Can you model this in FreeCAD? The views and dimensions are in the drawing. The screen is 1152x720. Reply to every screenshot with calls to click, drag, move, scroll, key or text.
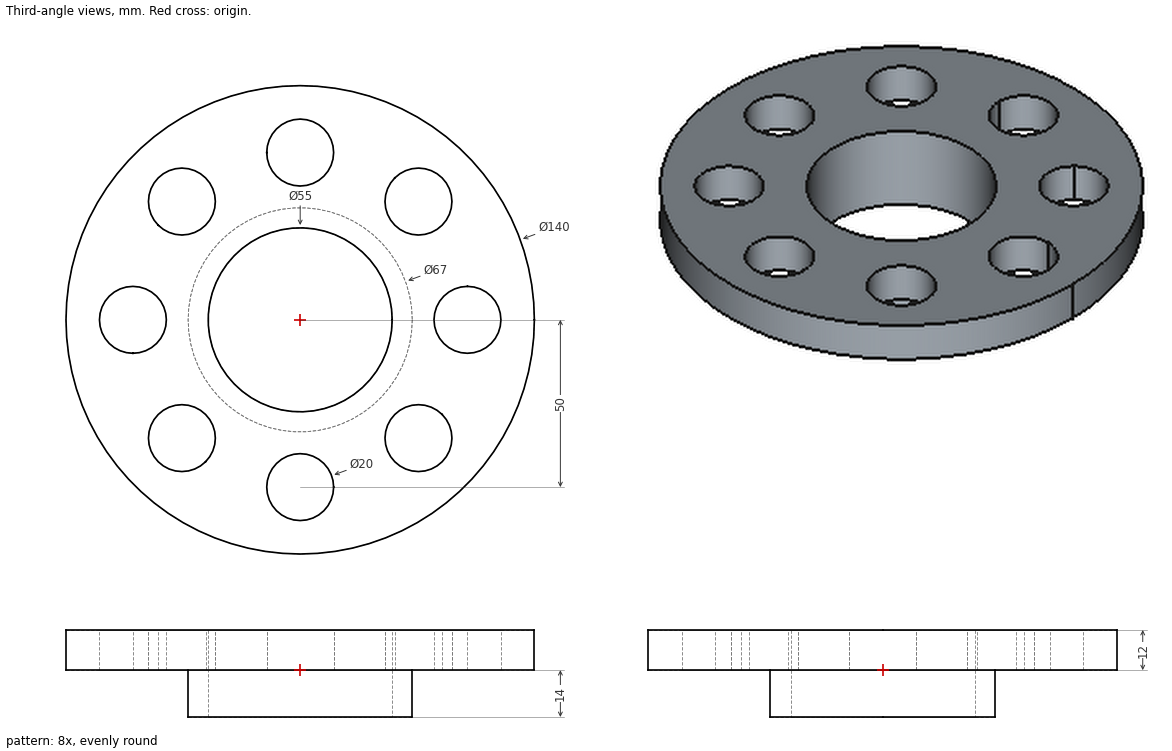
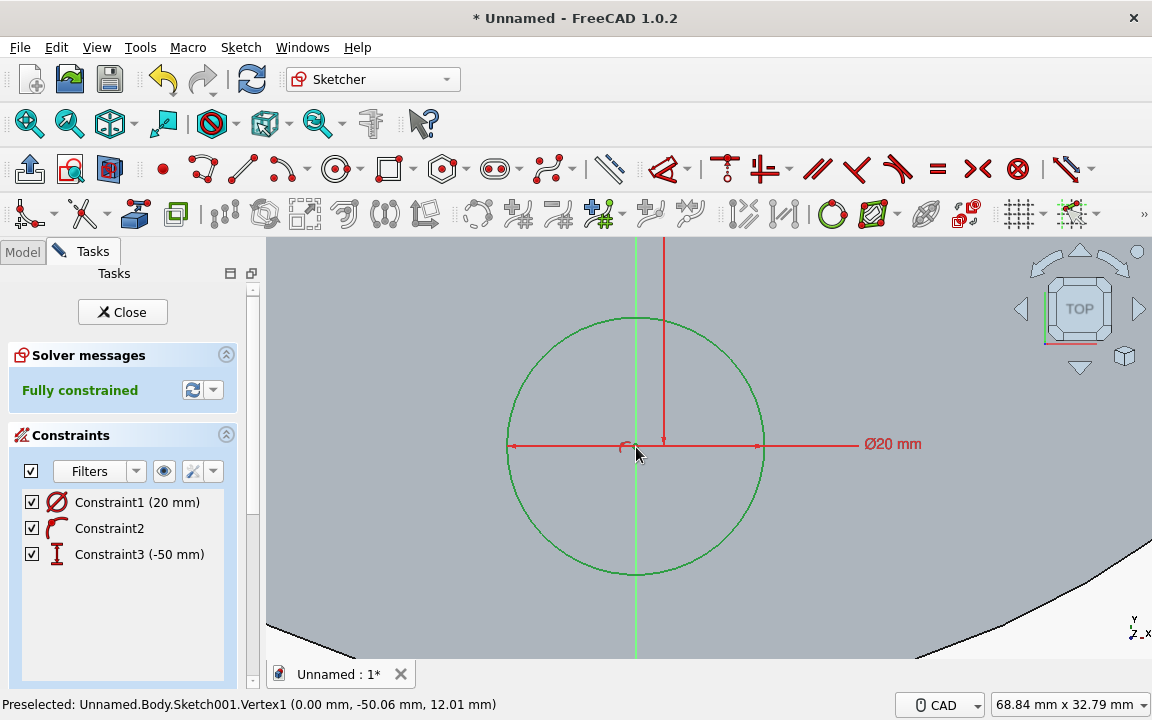
click(123, 312)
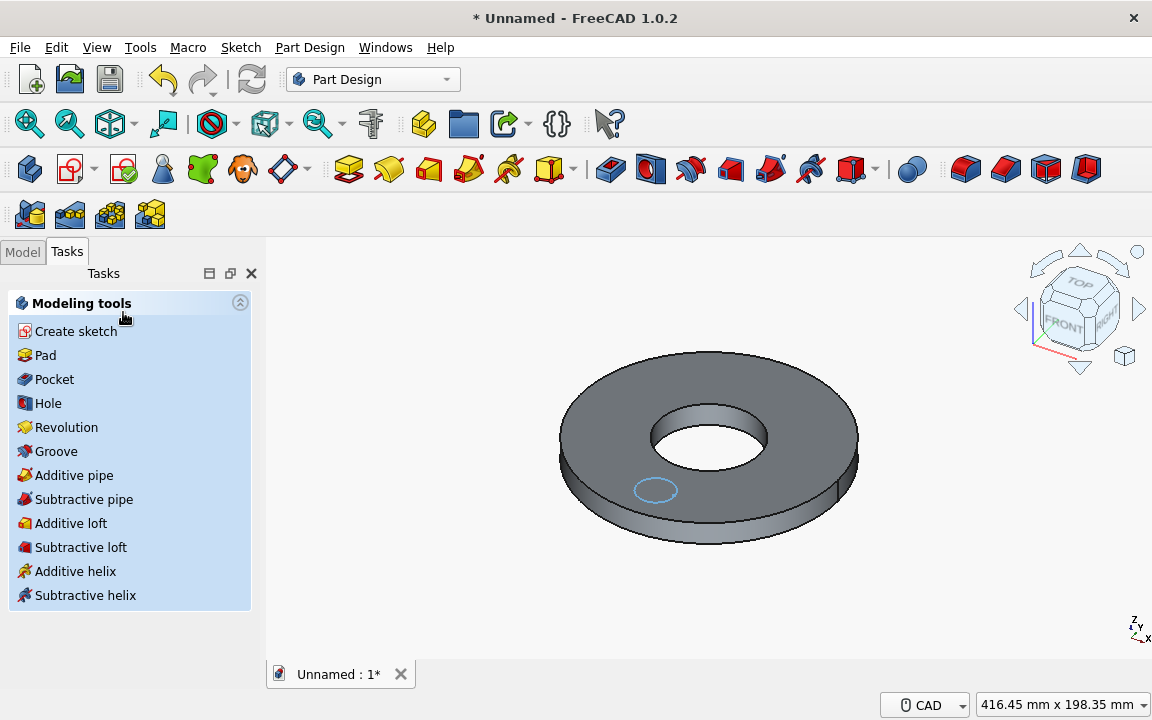
click(612, 170)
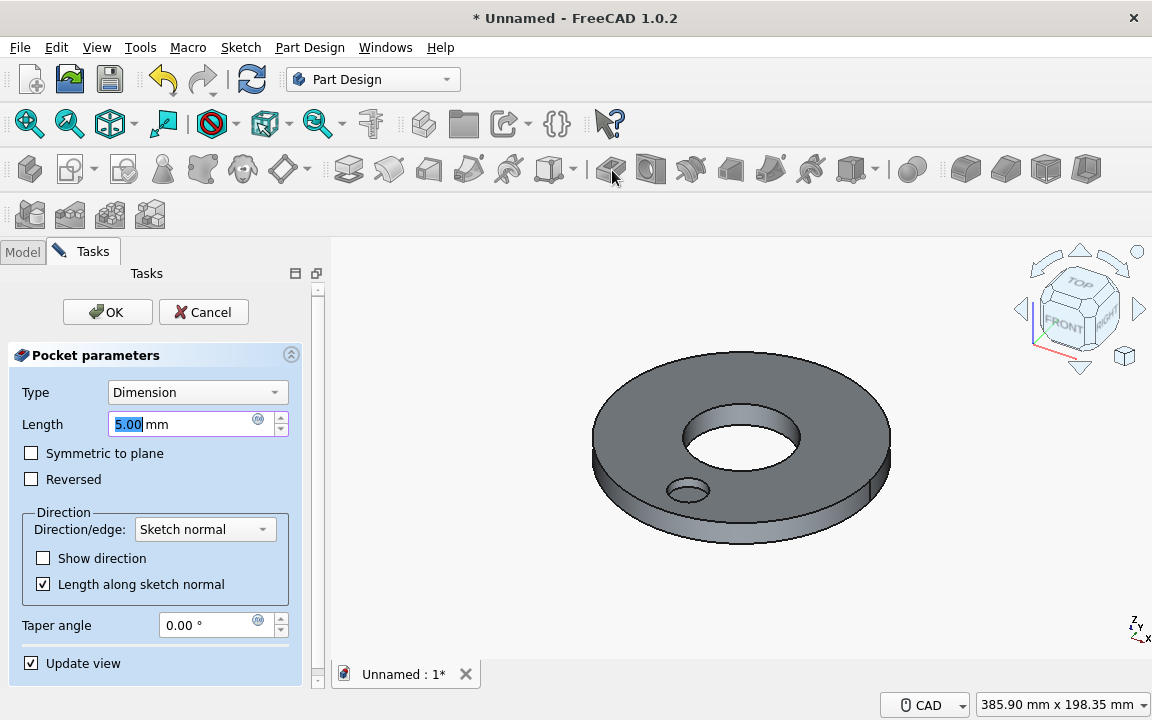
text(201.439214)
key(Tab)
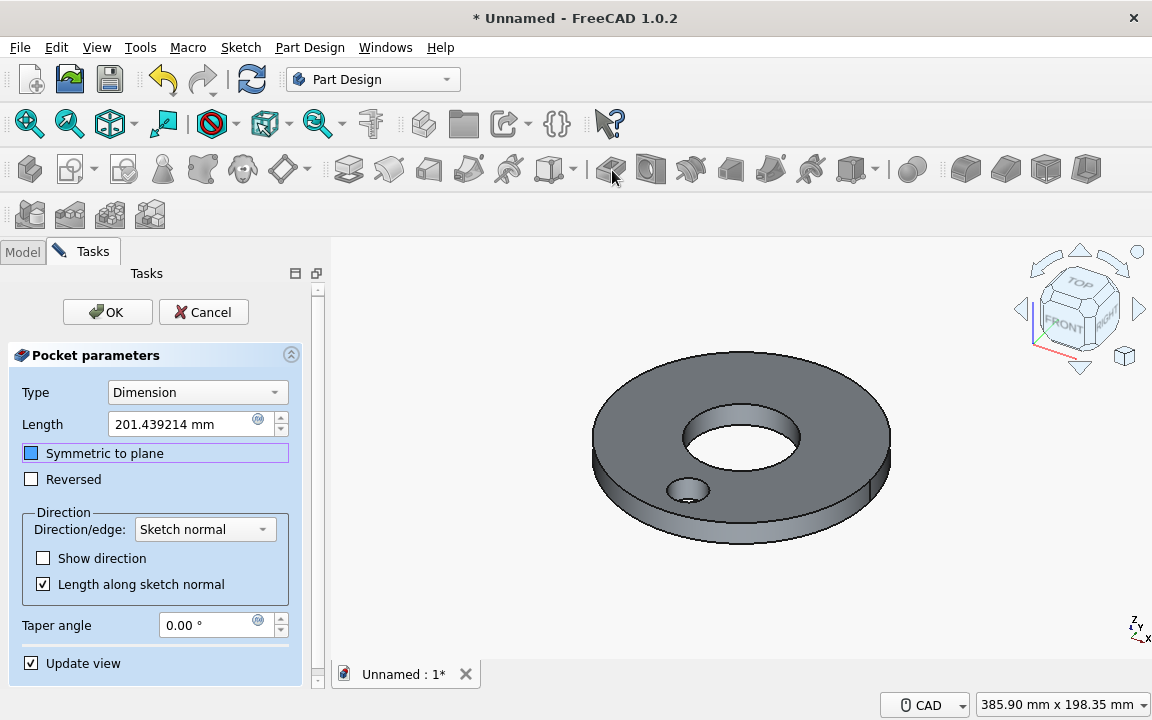
click(30, 453)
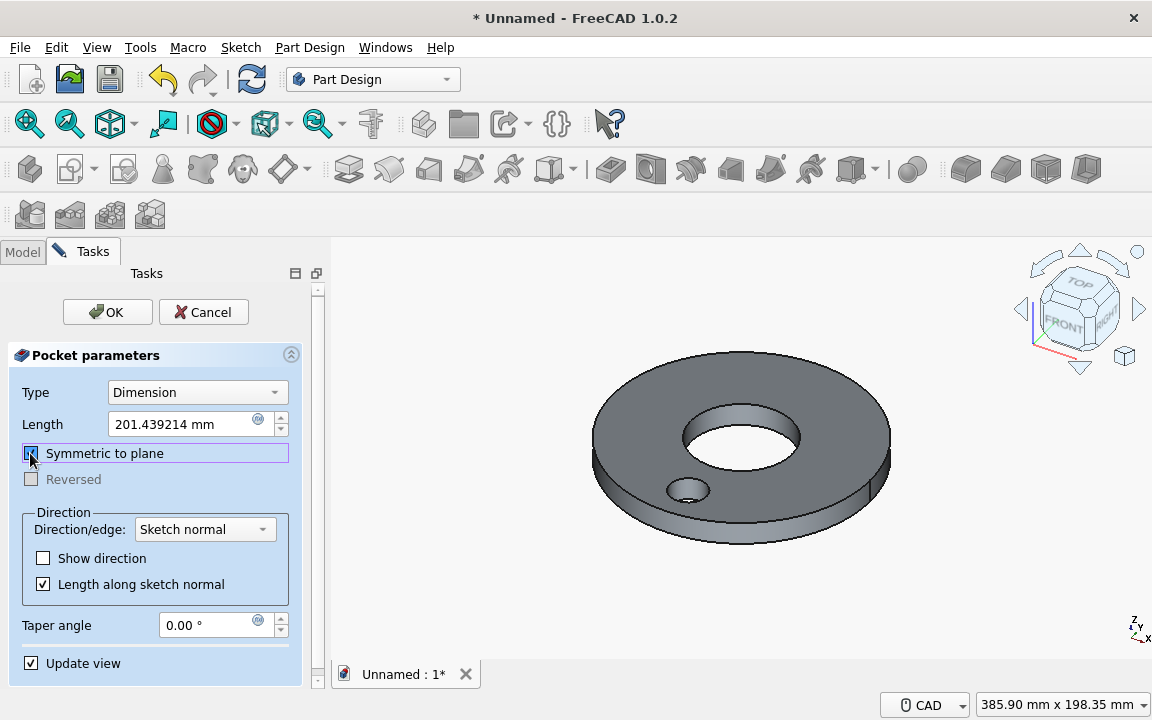
click(108, 312)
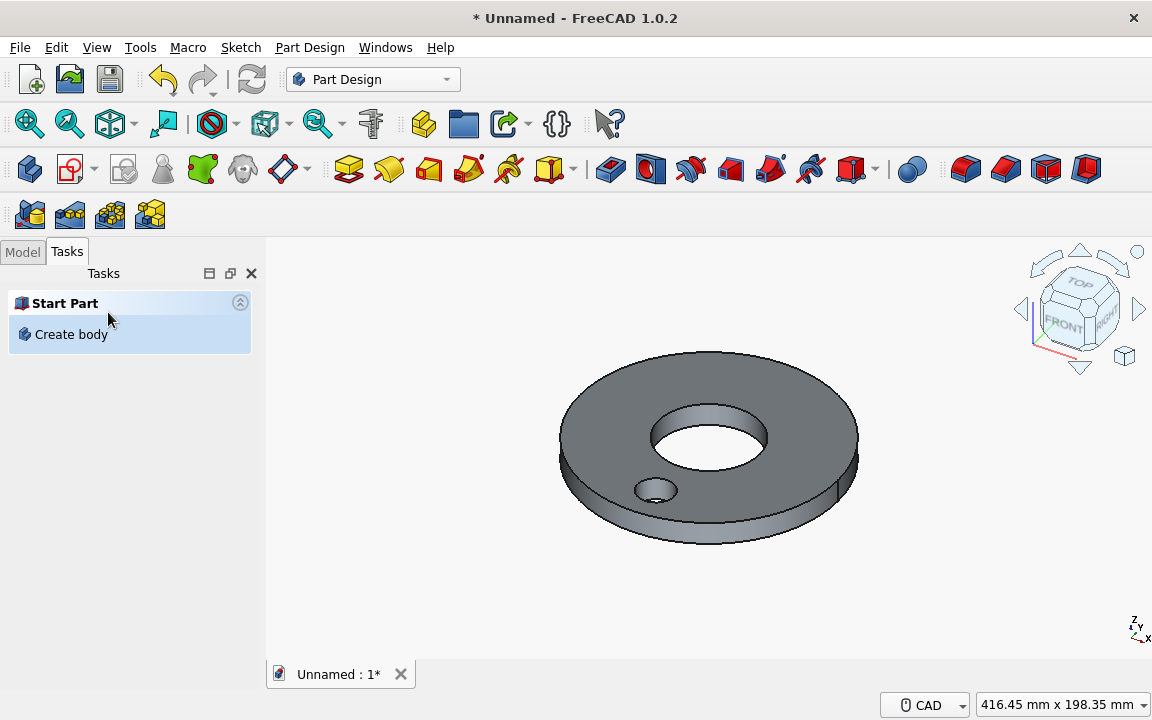
click(23, 251)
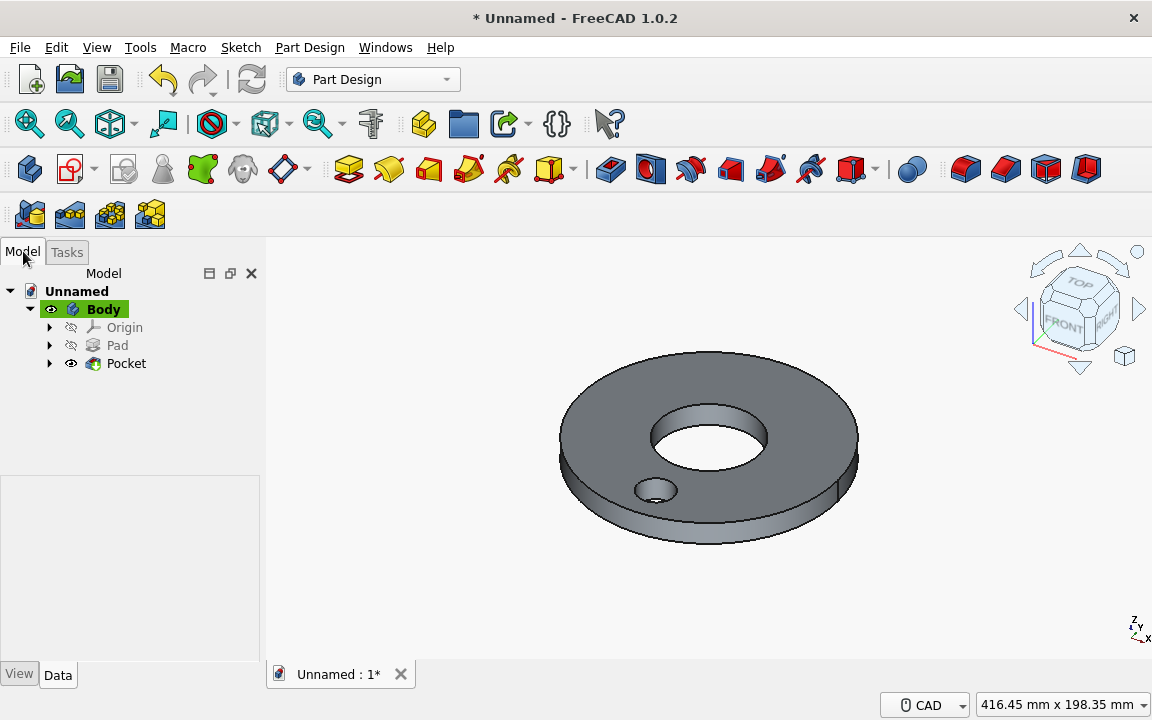
click(116, 363)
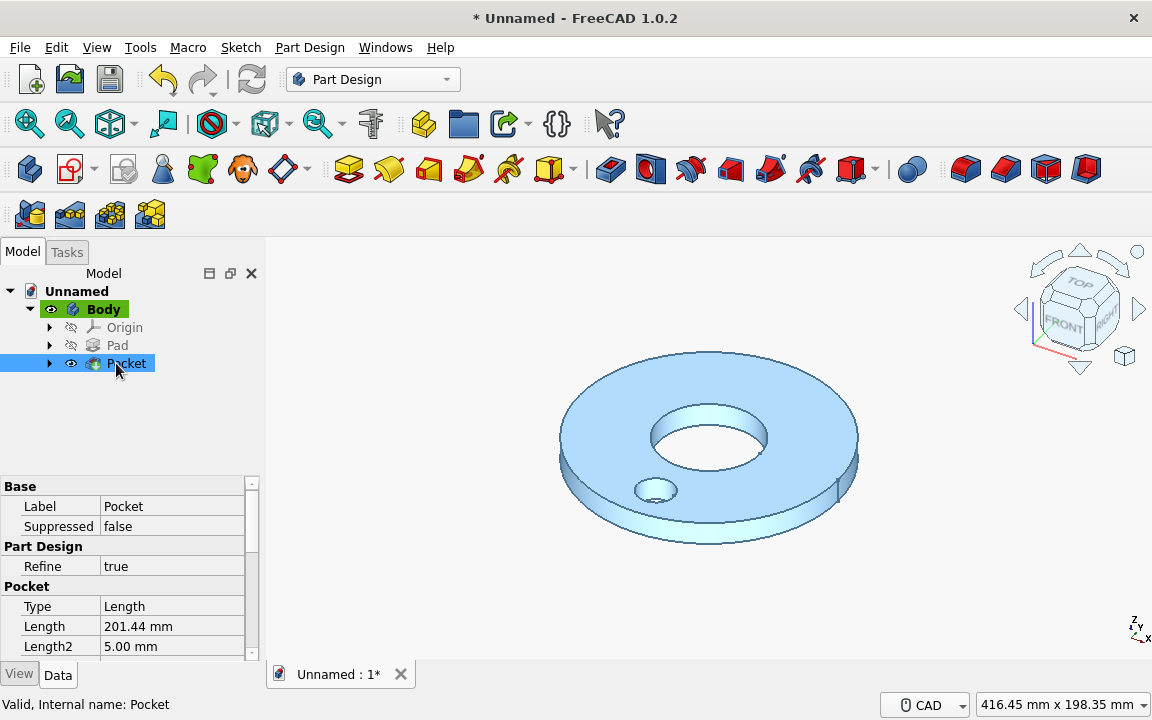
click(110, 214)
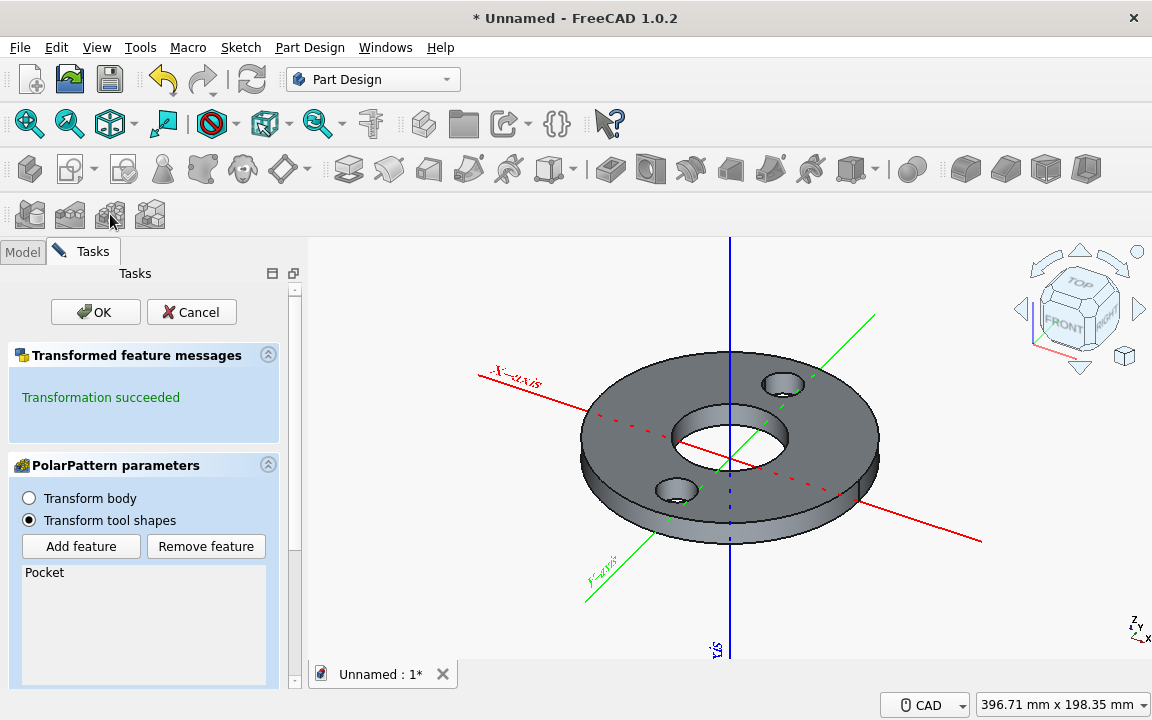
scroll(295, 486, down, 2)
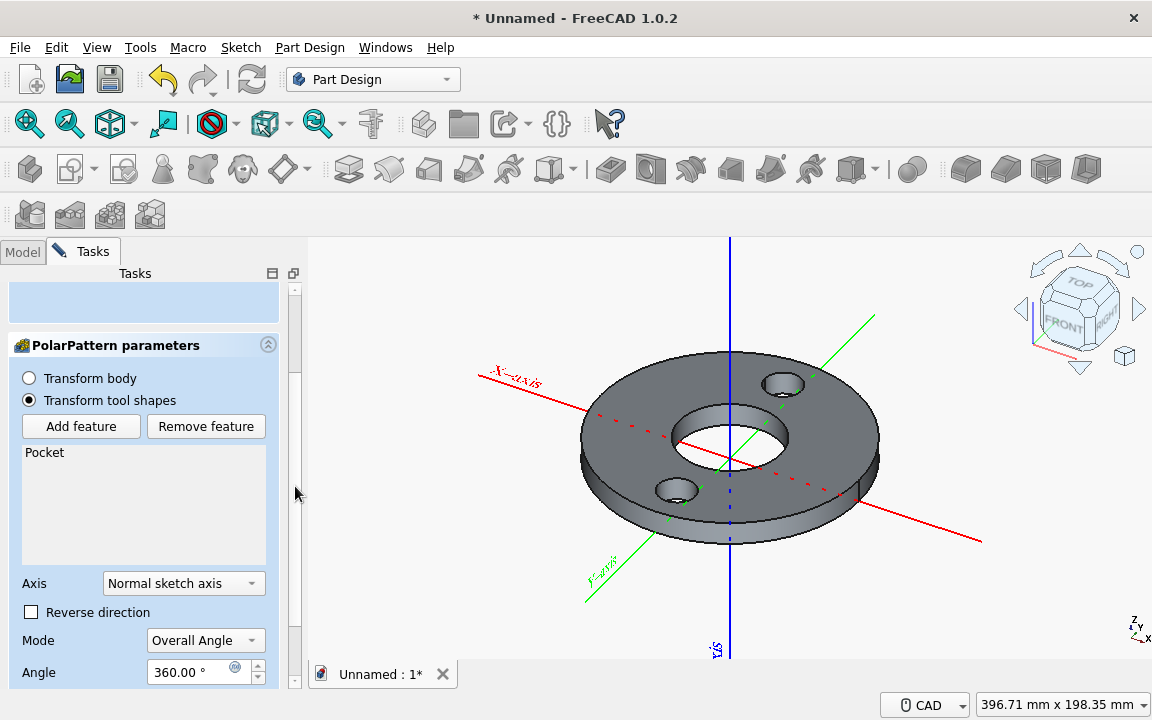
click(184, 584)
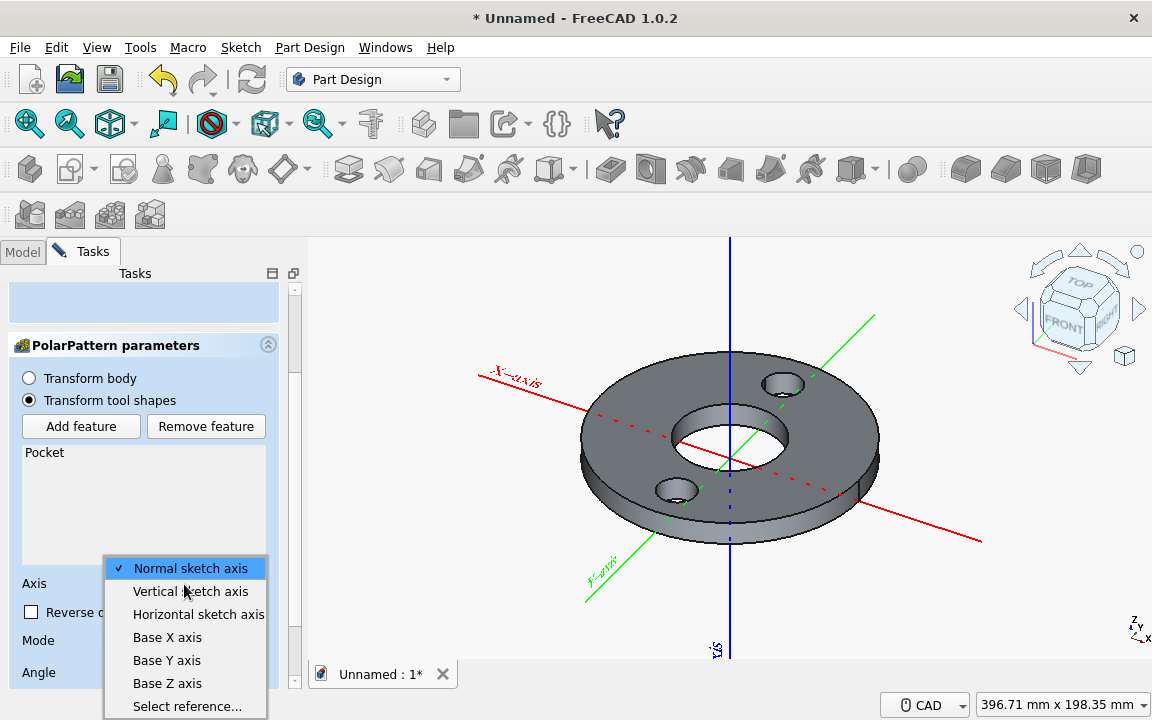
click(184, 684)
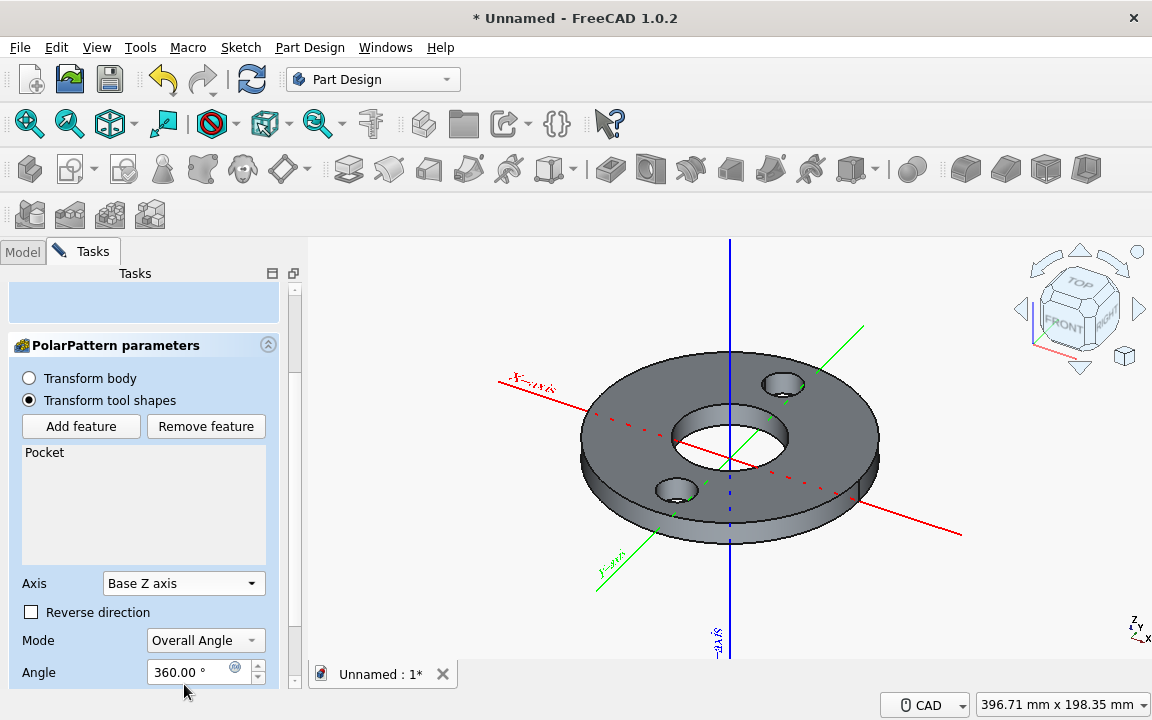
scroll(295, 486, down, 2)